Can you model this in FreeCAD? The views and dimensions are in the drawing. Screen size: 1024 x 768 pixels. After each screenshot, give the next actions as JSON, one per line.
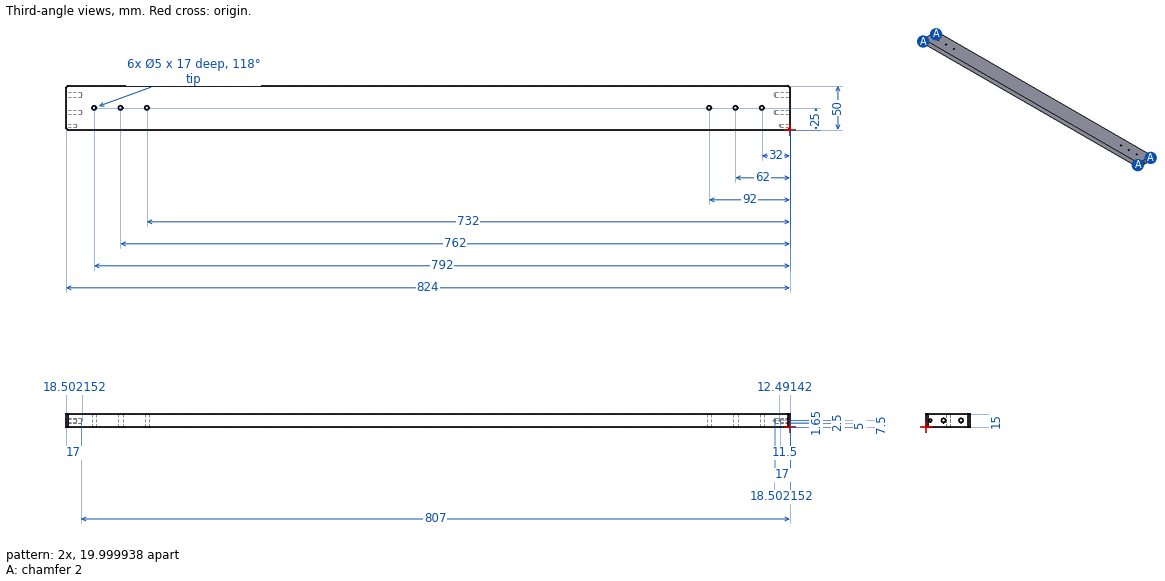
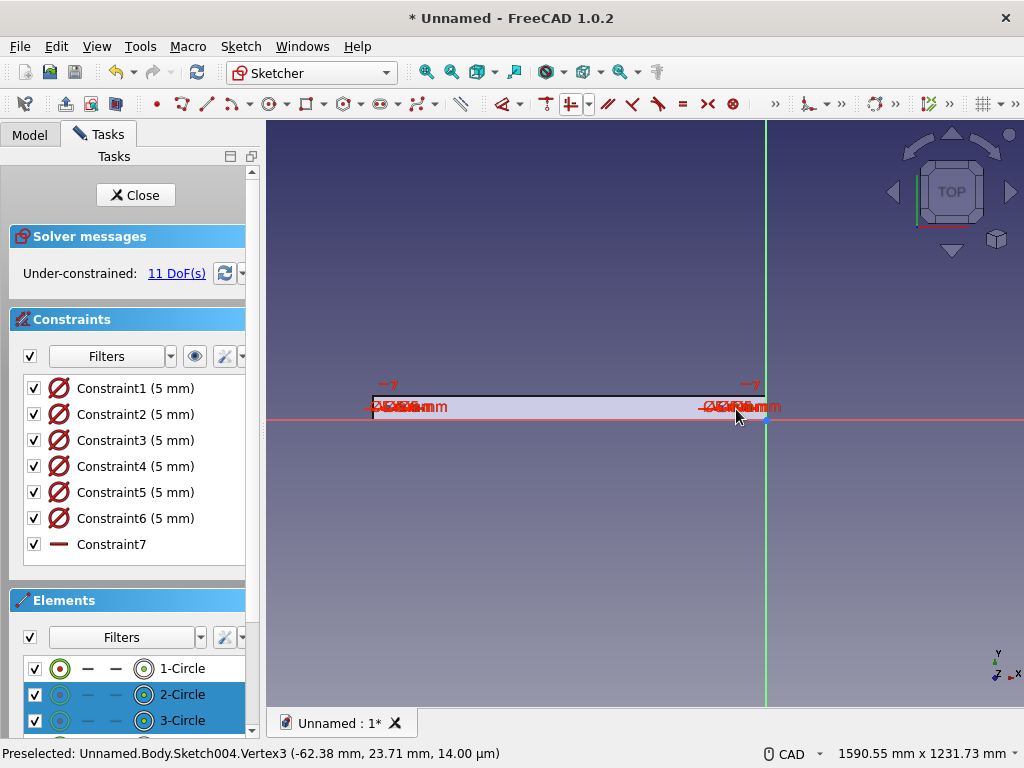
{"action": "key", "text": "h"}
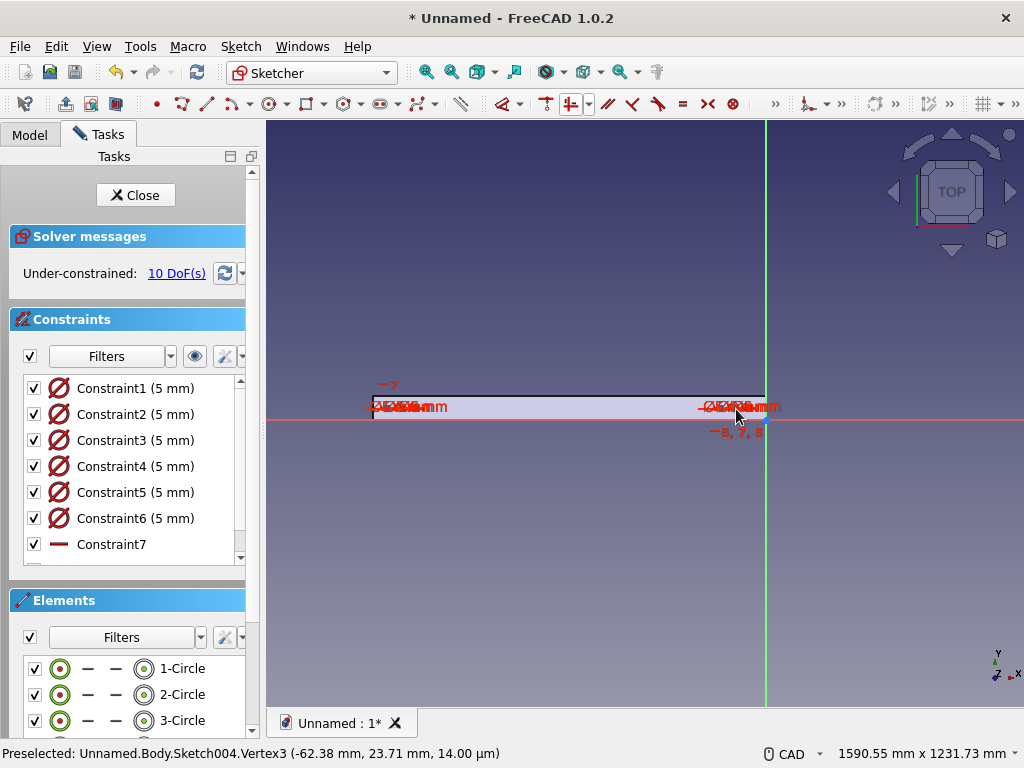
{"action": "left_click", "coordinate": [736, 409]}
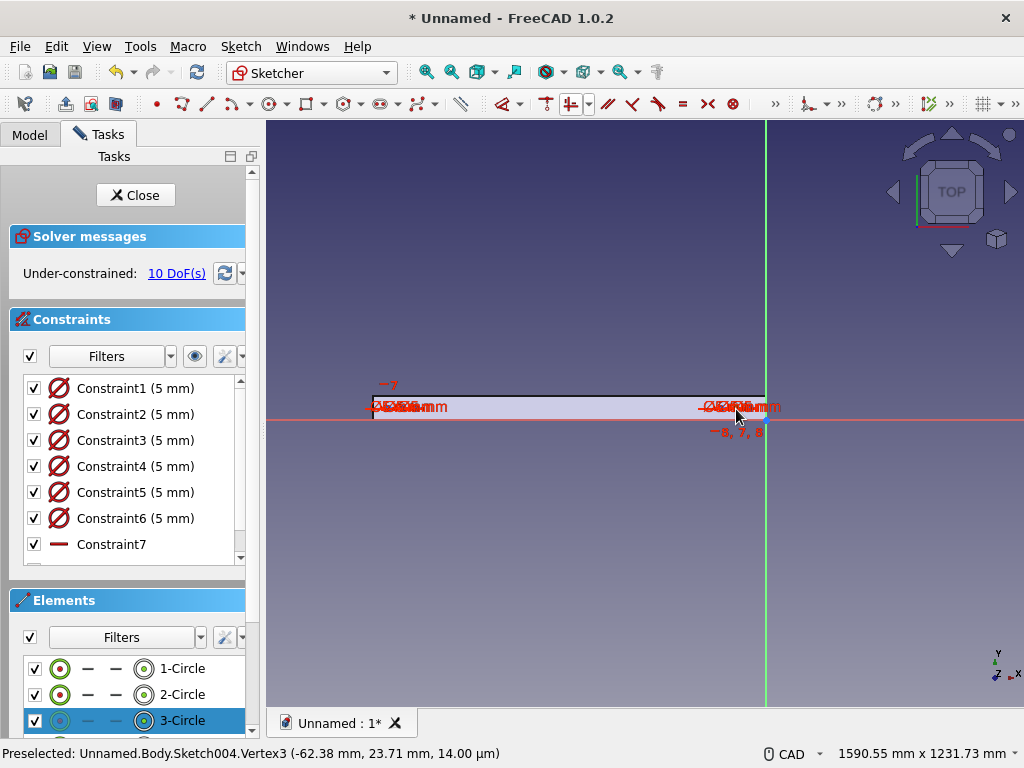
{"action": "left_click", "coordinate": [722, 409]}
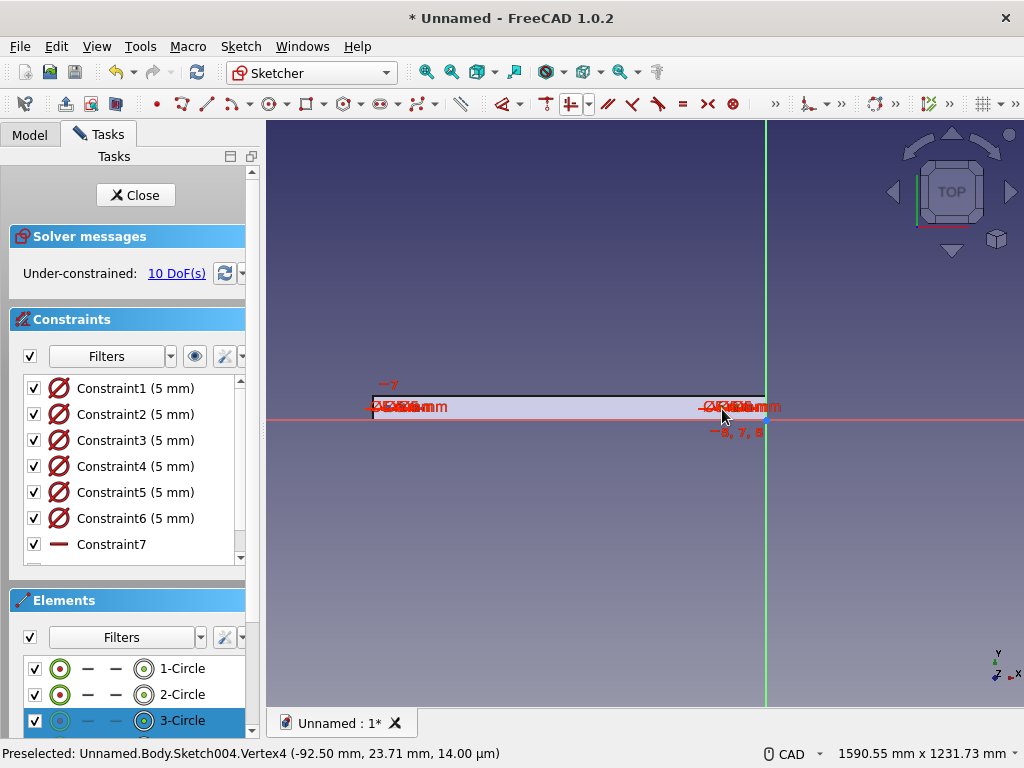
{"action": "key", "text": "h"}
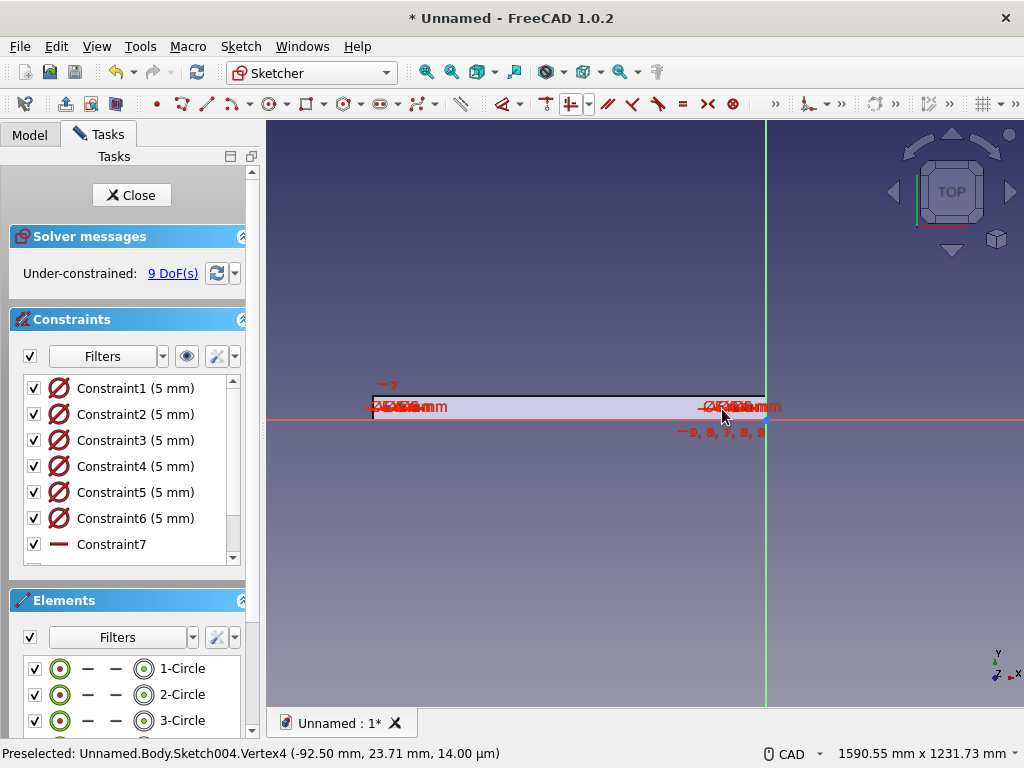
{"action": "left_click", "coordinate": [389, 409]}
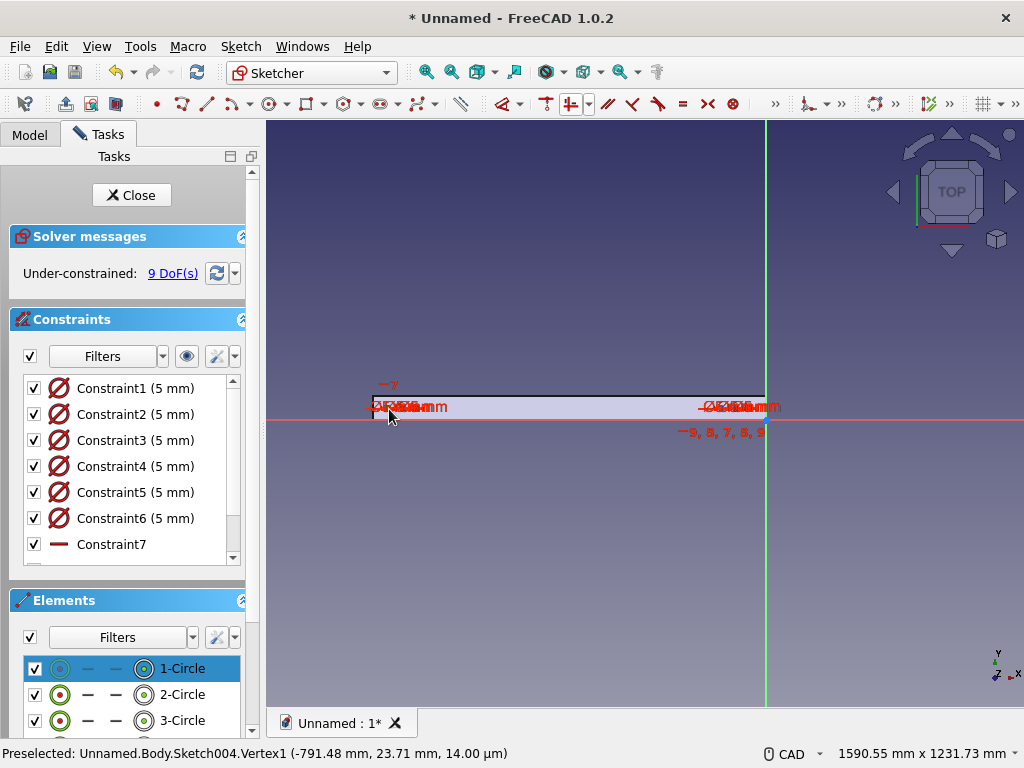
{"action": "left_click", "coordinate": [417, 409]}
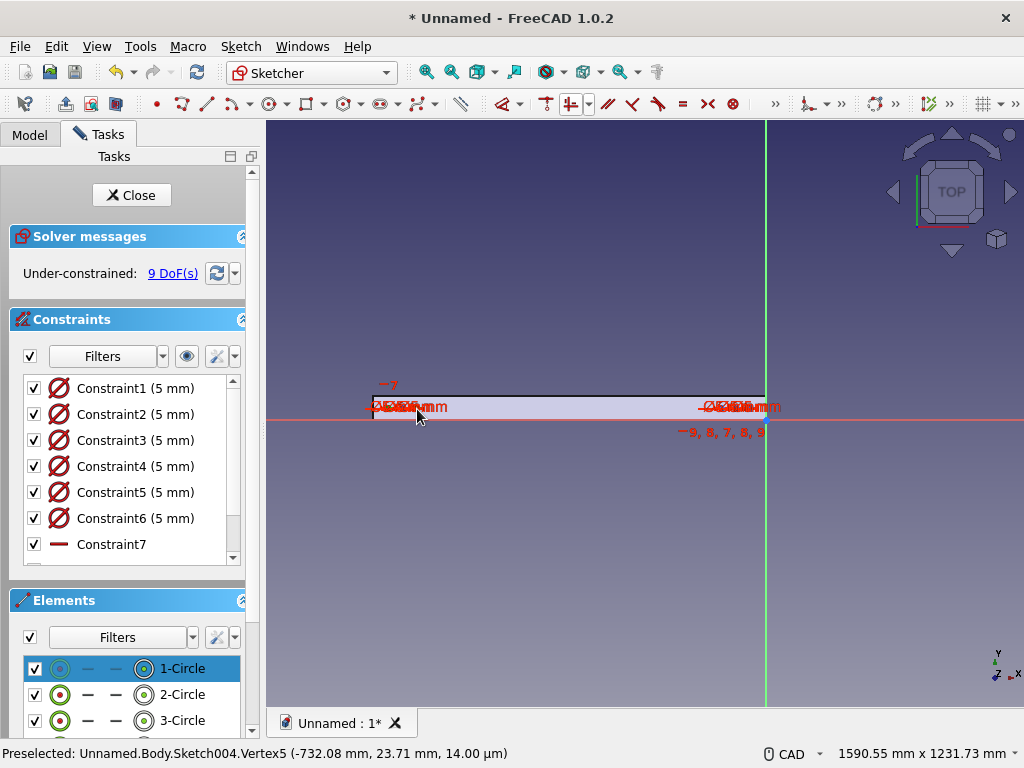
{"action": "key", "text": "h"}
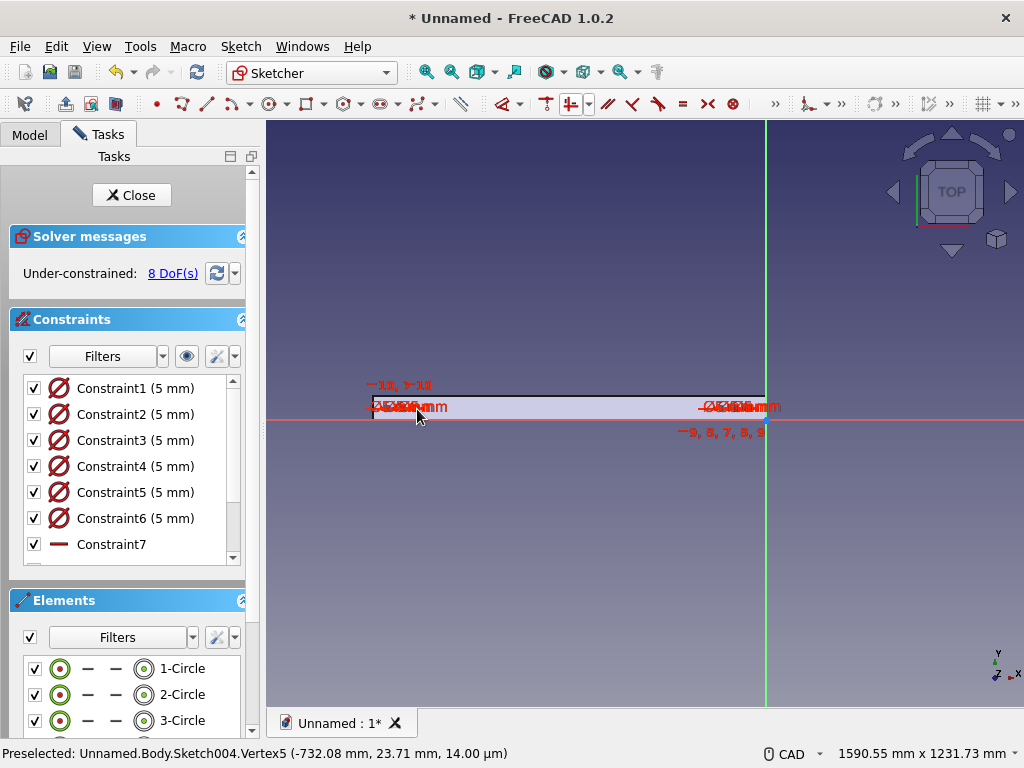
{"action": "left_click", "coordinate": [389, 409]}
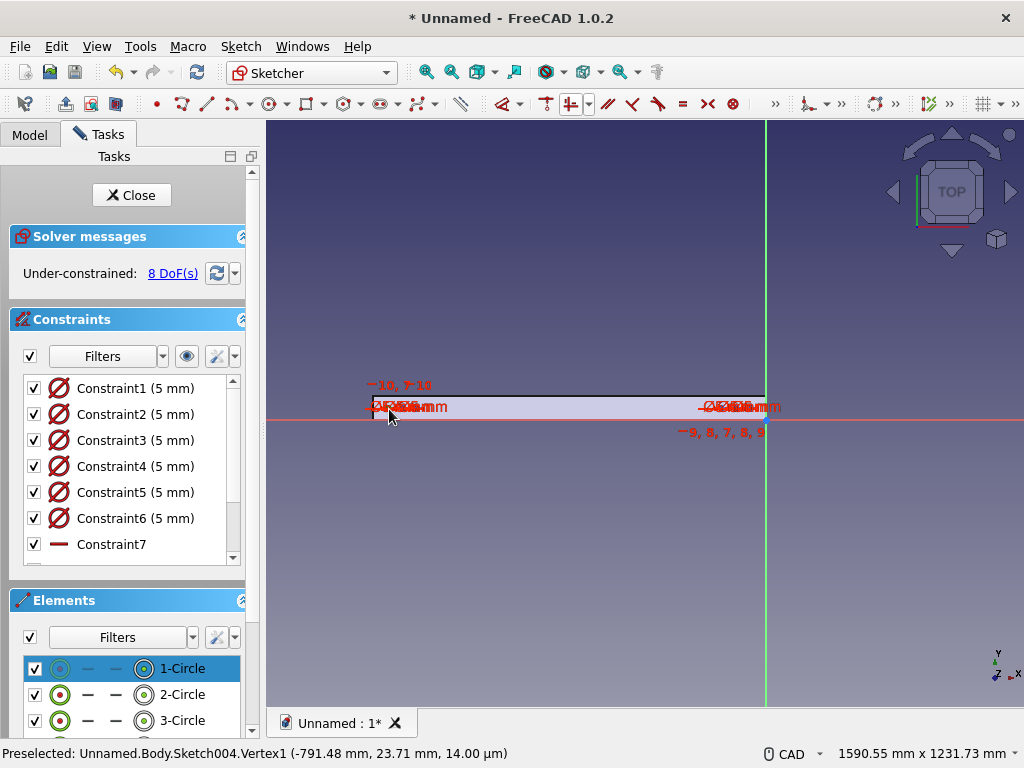
{"action": "left_click", "coordinate": [403, 409]}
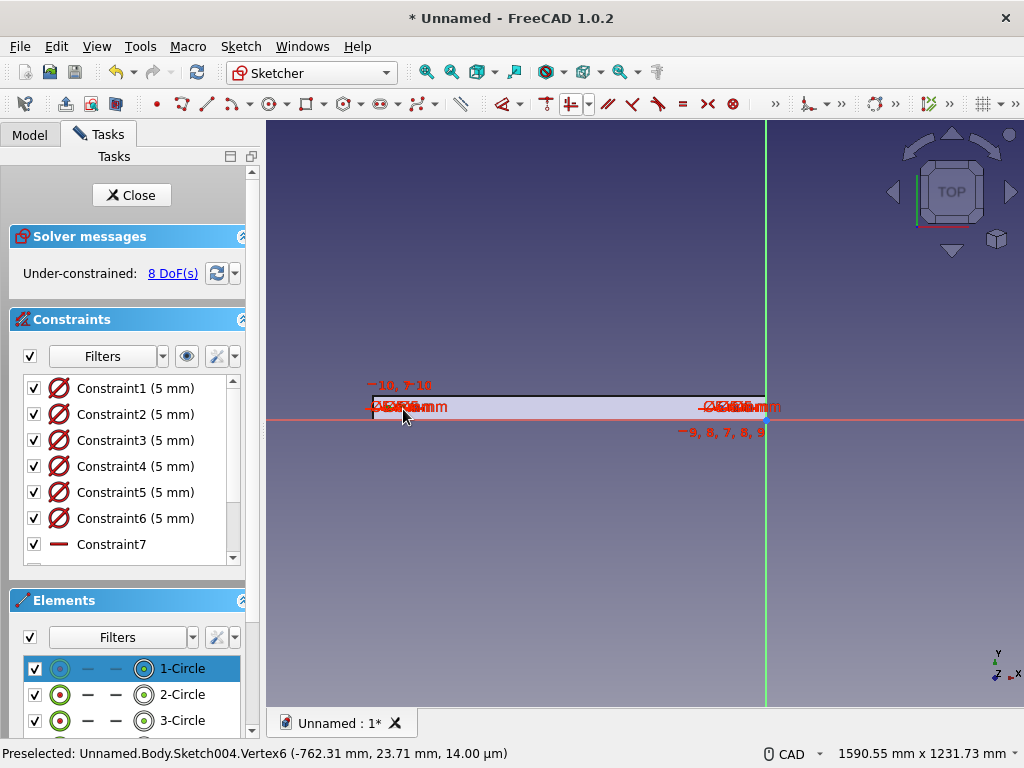
{"action": "key", "text": "h"}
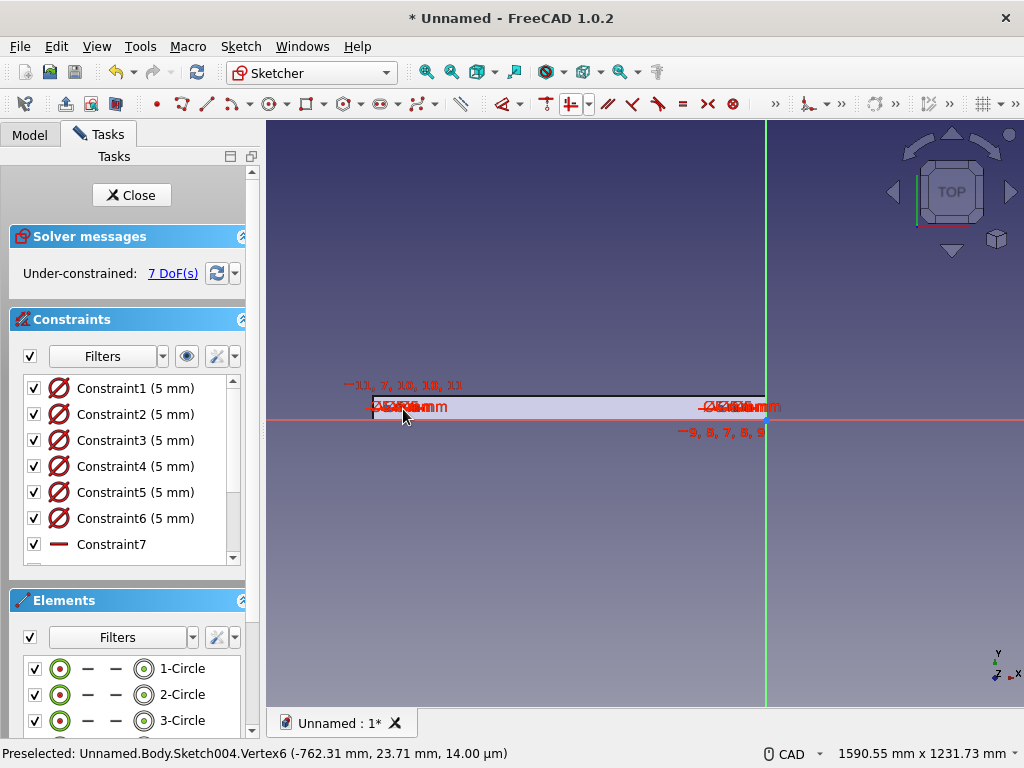
{"action": "left_click", "coordinate": [502, 104]}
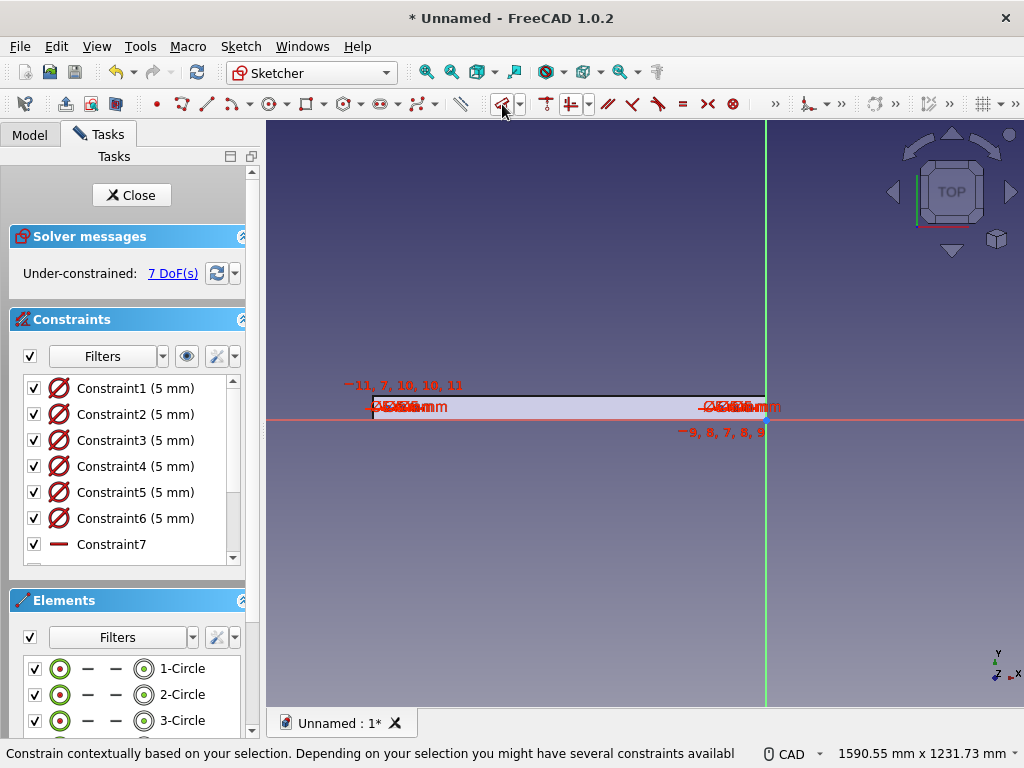
{"action": "scroll", "coordinate": [389, 409], "scroll_direction": "up", "scroll_amount": 7}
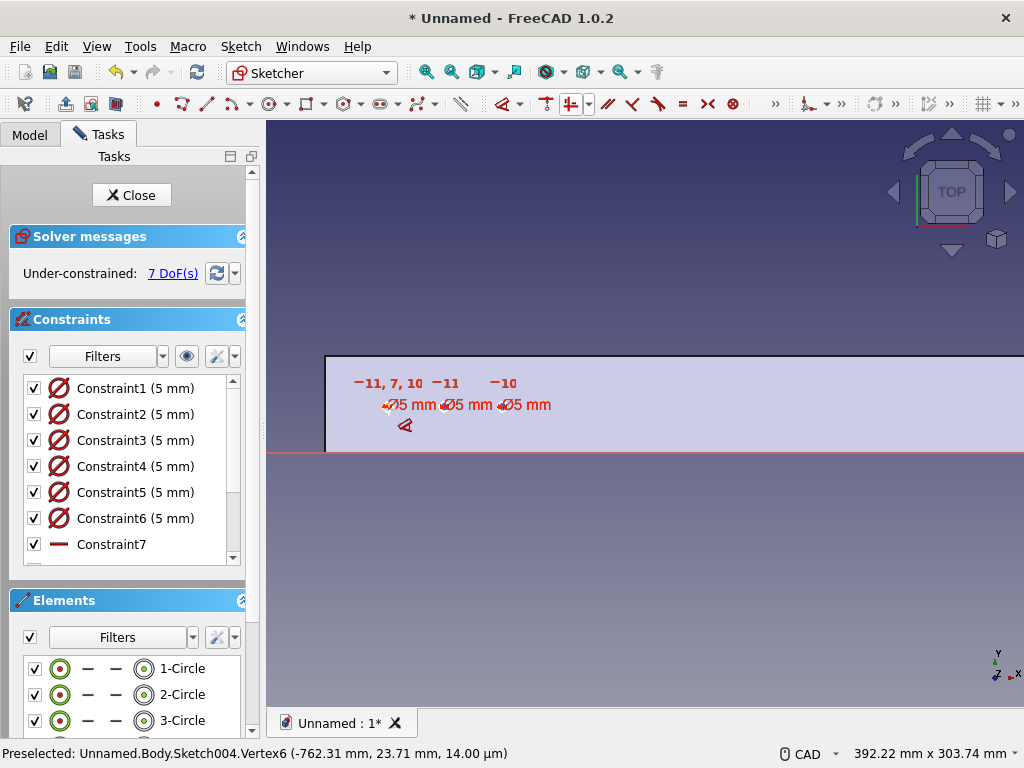
{"action": "left_click", "coordinate": [388, 407]}
{"action": "left_click", "coordinate": [354, 430]}